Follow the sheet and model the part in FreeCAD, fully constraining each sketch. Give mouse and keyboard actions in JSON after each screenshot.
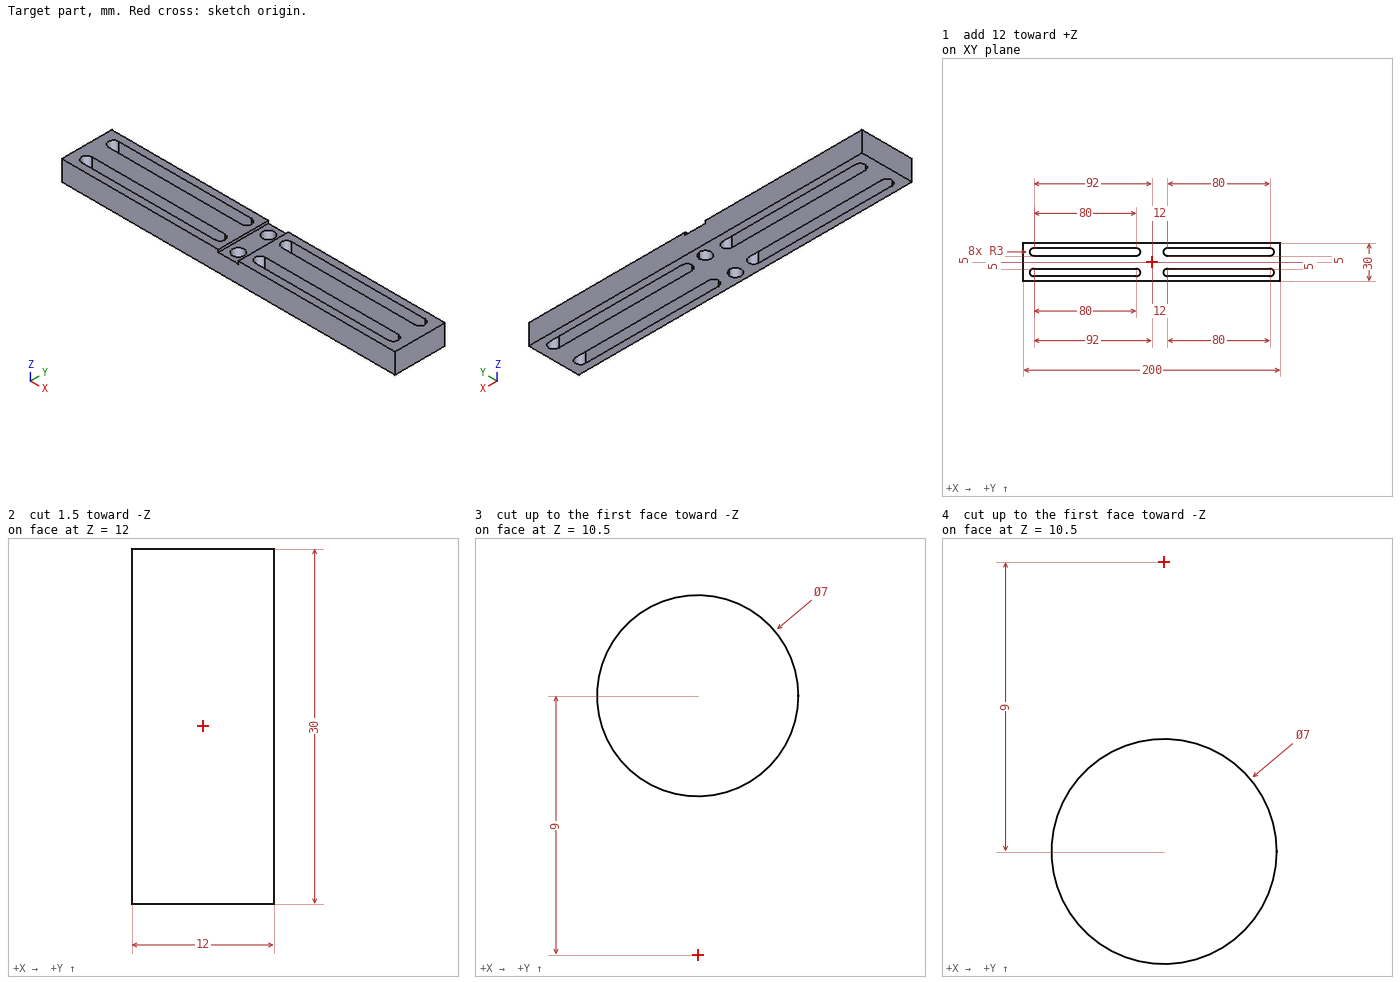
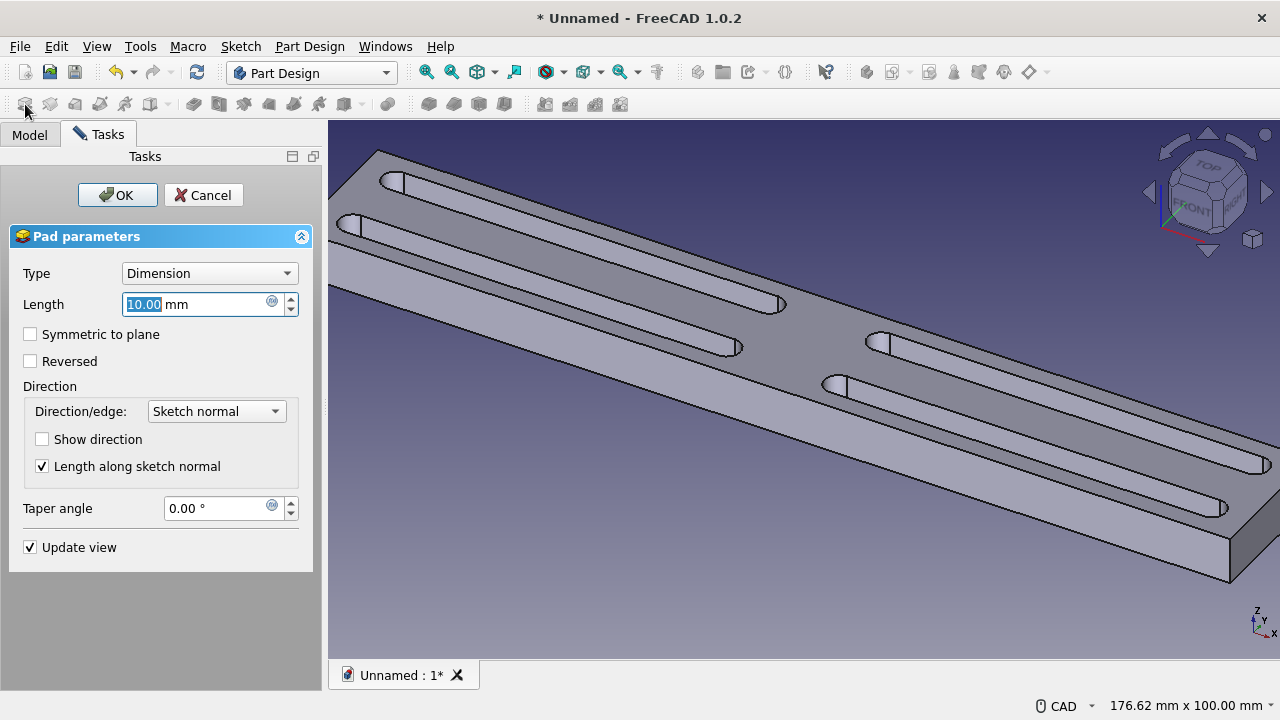
{"action": "type", "text": "12"}
{"action": "key", "text": "Tab"}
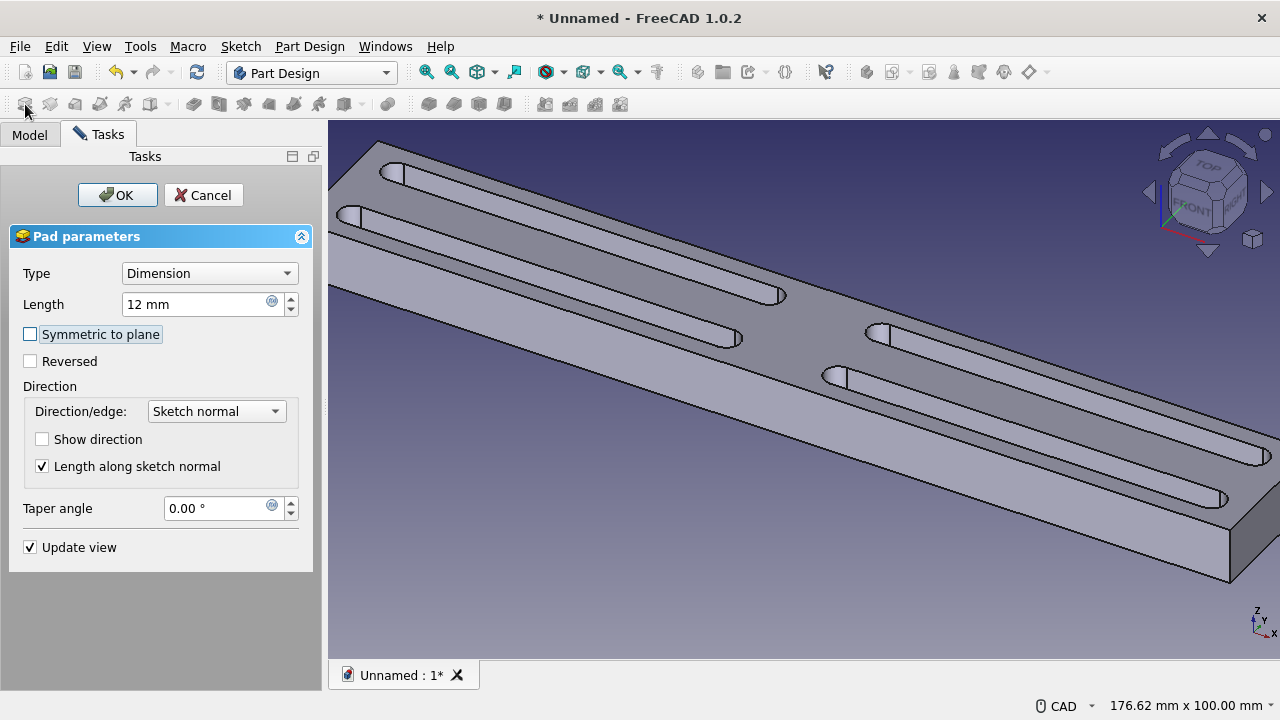
{"action": "left_click", "coordinate": [118, 195]}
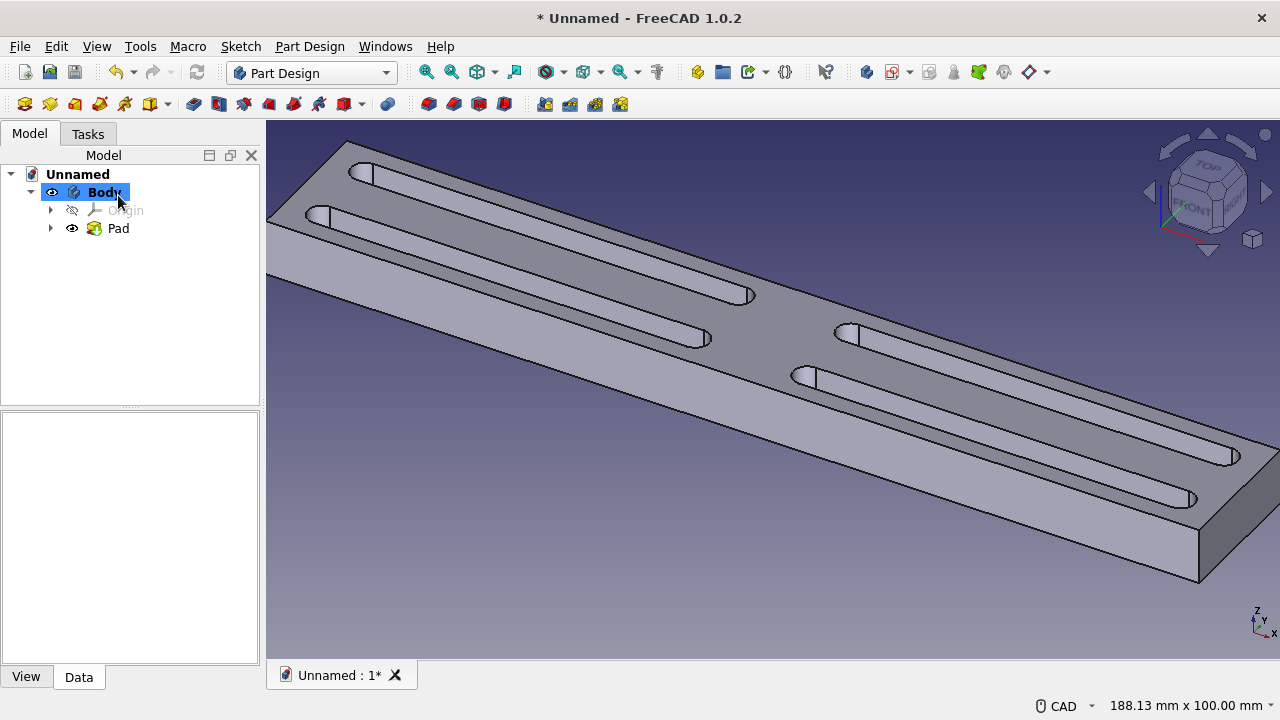
{"action": "left_click", "coordinate": [773, 335]}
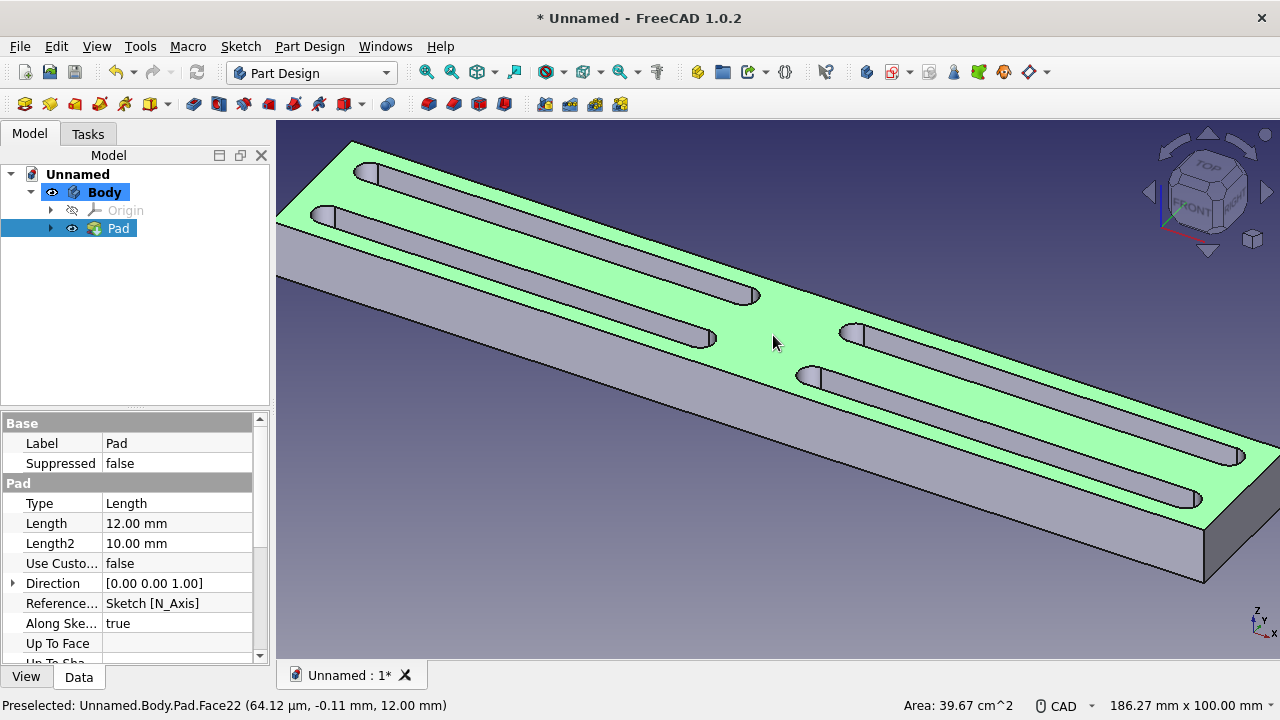
{"action": "left_click", "coordinate": [892, 72]}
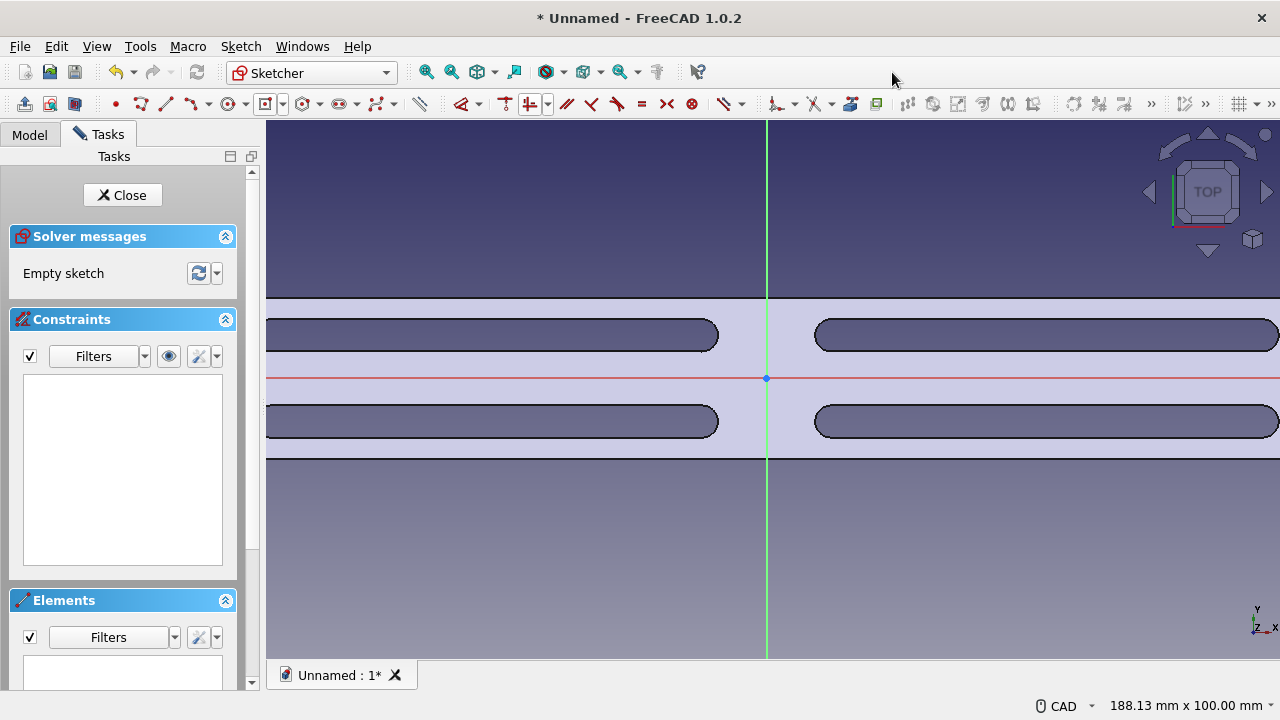
{"action": "scroll", "coordinate": [817, 369], "scroll_direction": "up", "scroll_amount": 4}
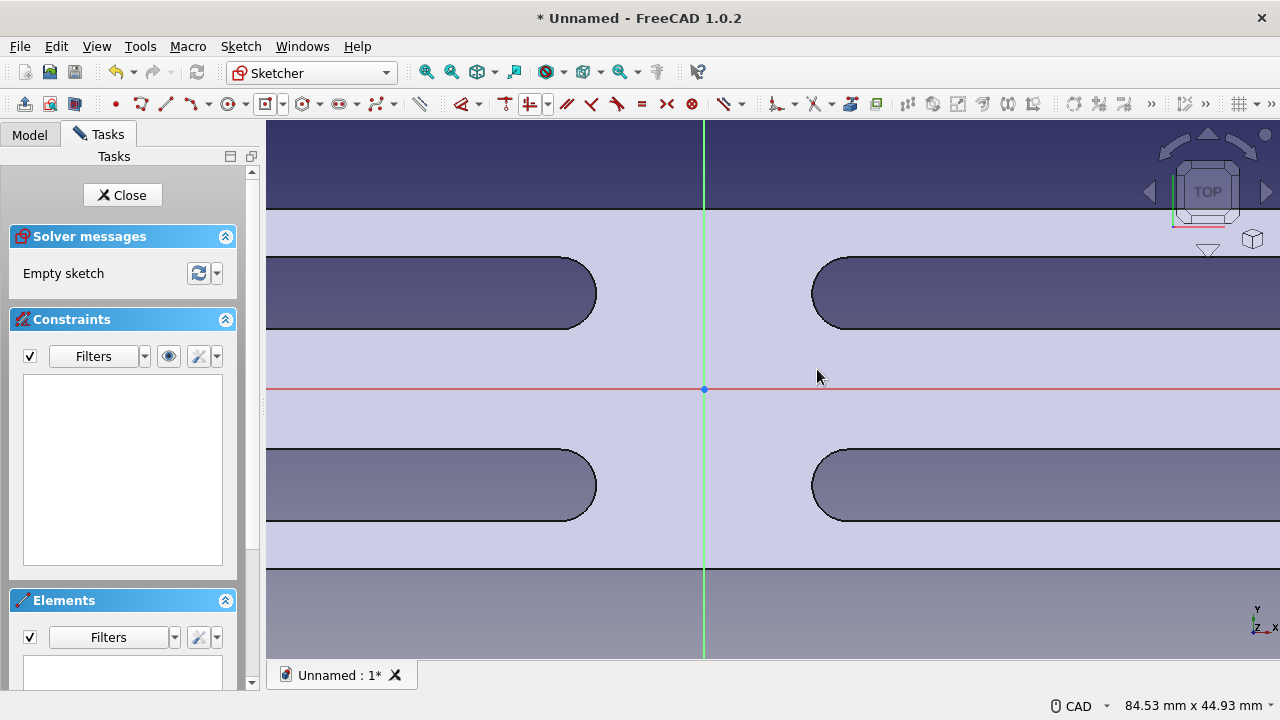
{"action": "left_click", "coordinate": [264, 104]}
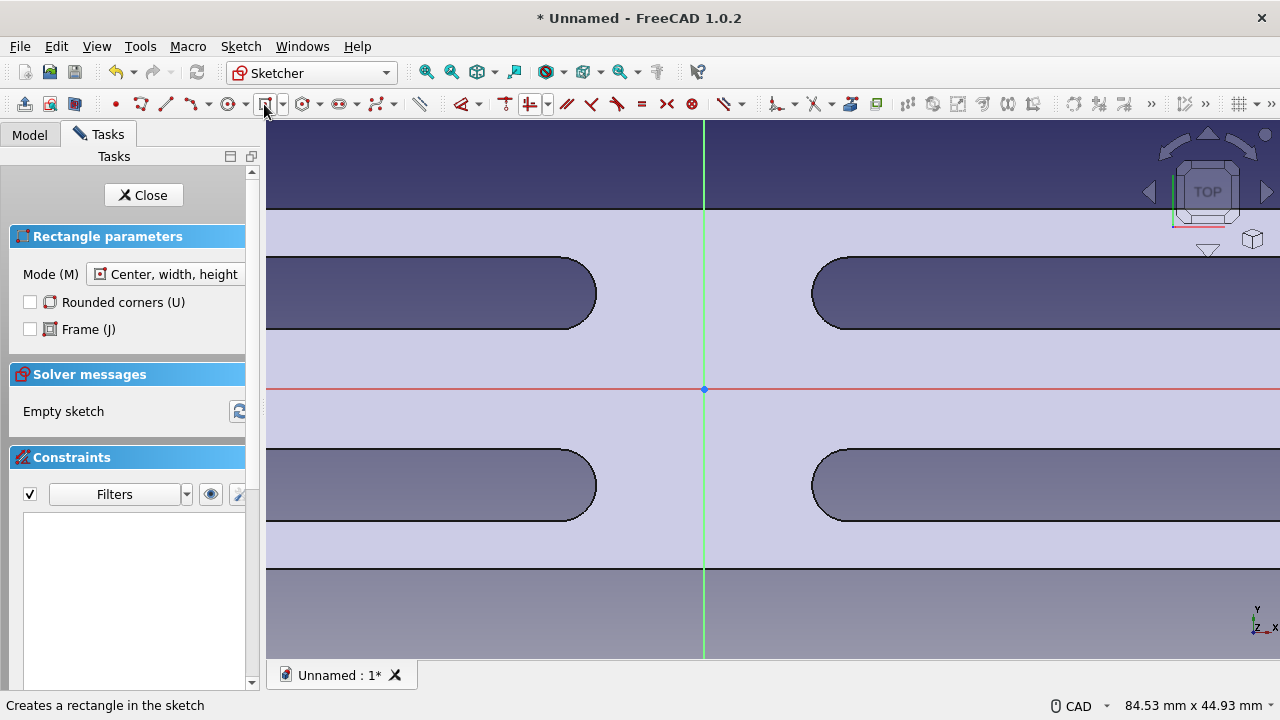
{"action": "left_click", "coordinate": [704, 389]}
{"action": "mouse_move", "coordinate": [776, 209]}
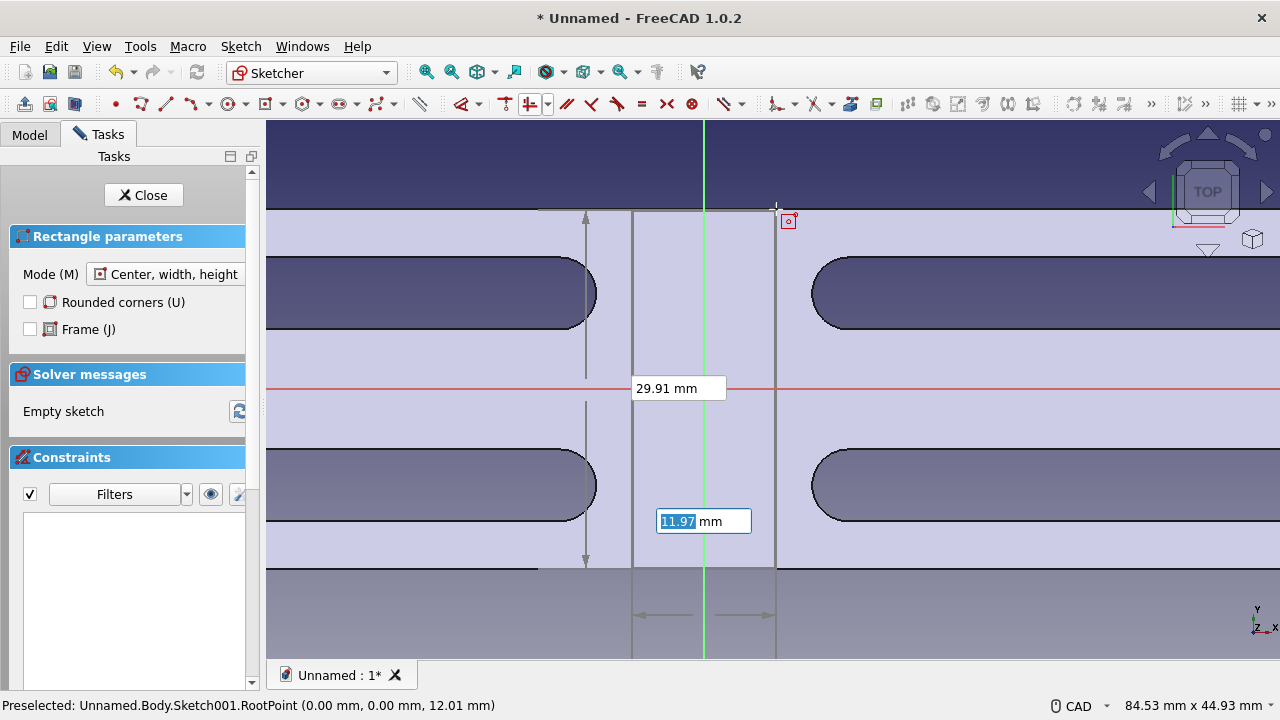
{"action": "type", "text": "12"}
{"action": "key", "text": "Tab"}
{"action": "type", "text": "30"}
{"action": "key", "text": "Return"}
{"action": "key", "text": "Escape"}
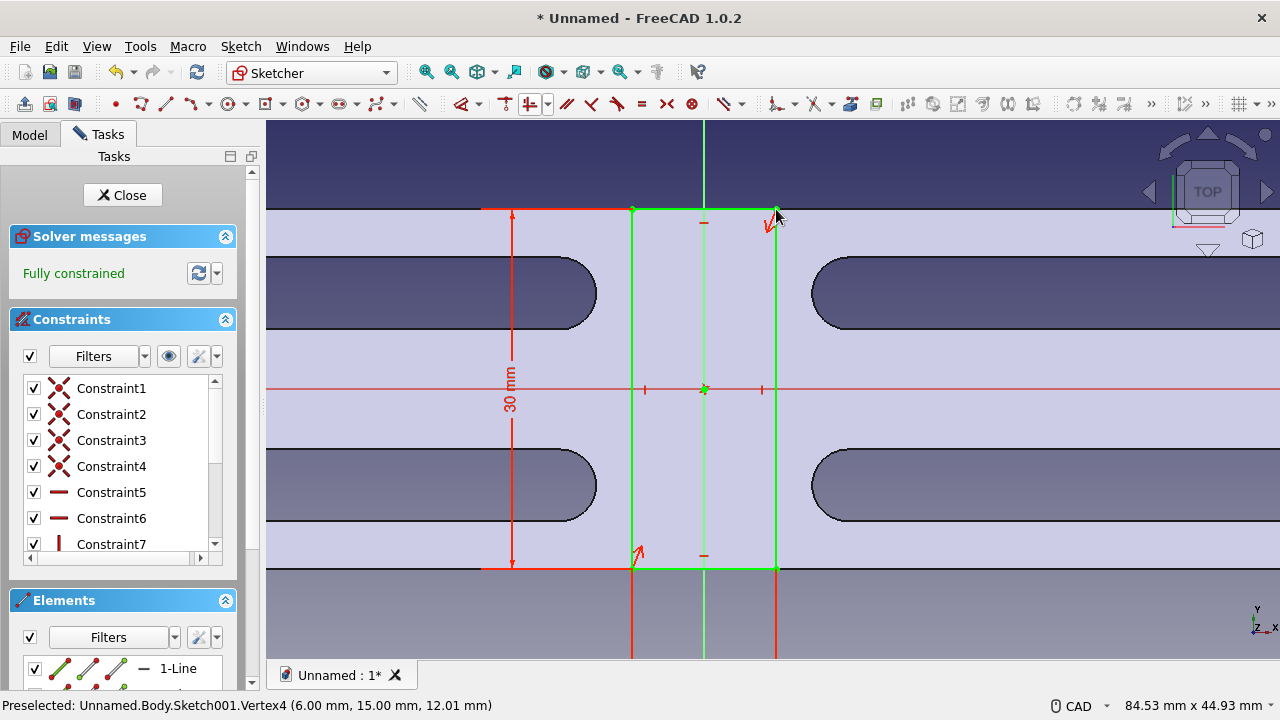
{"action": "left_click", "coordinate": [123, 195]}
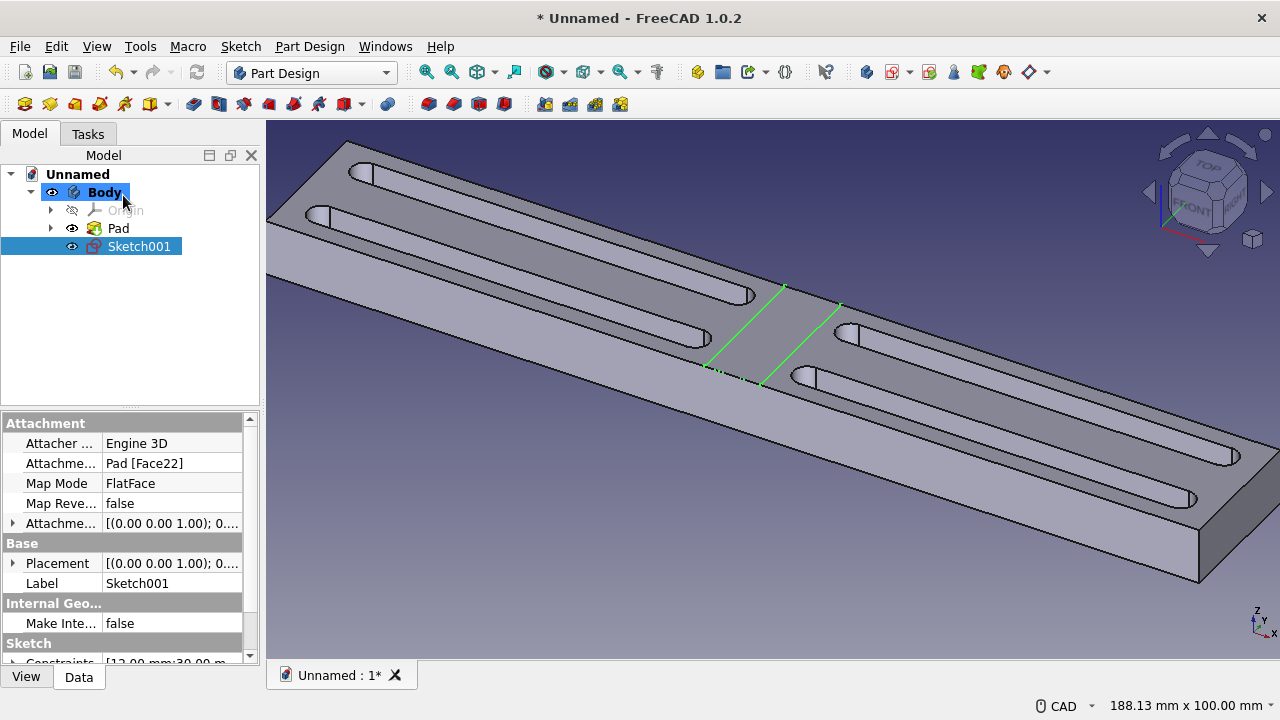
{"action": "left_click", "coordinate": [194, 104]}